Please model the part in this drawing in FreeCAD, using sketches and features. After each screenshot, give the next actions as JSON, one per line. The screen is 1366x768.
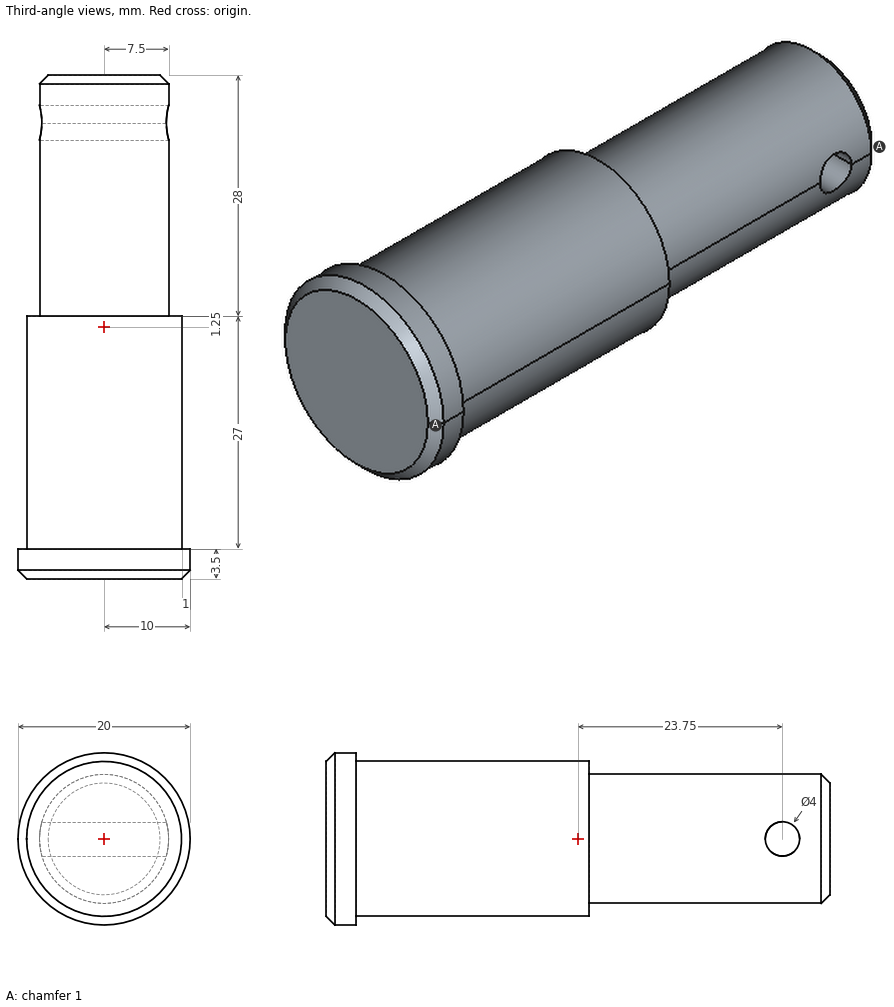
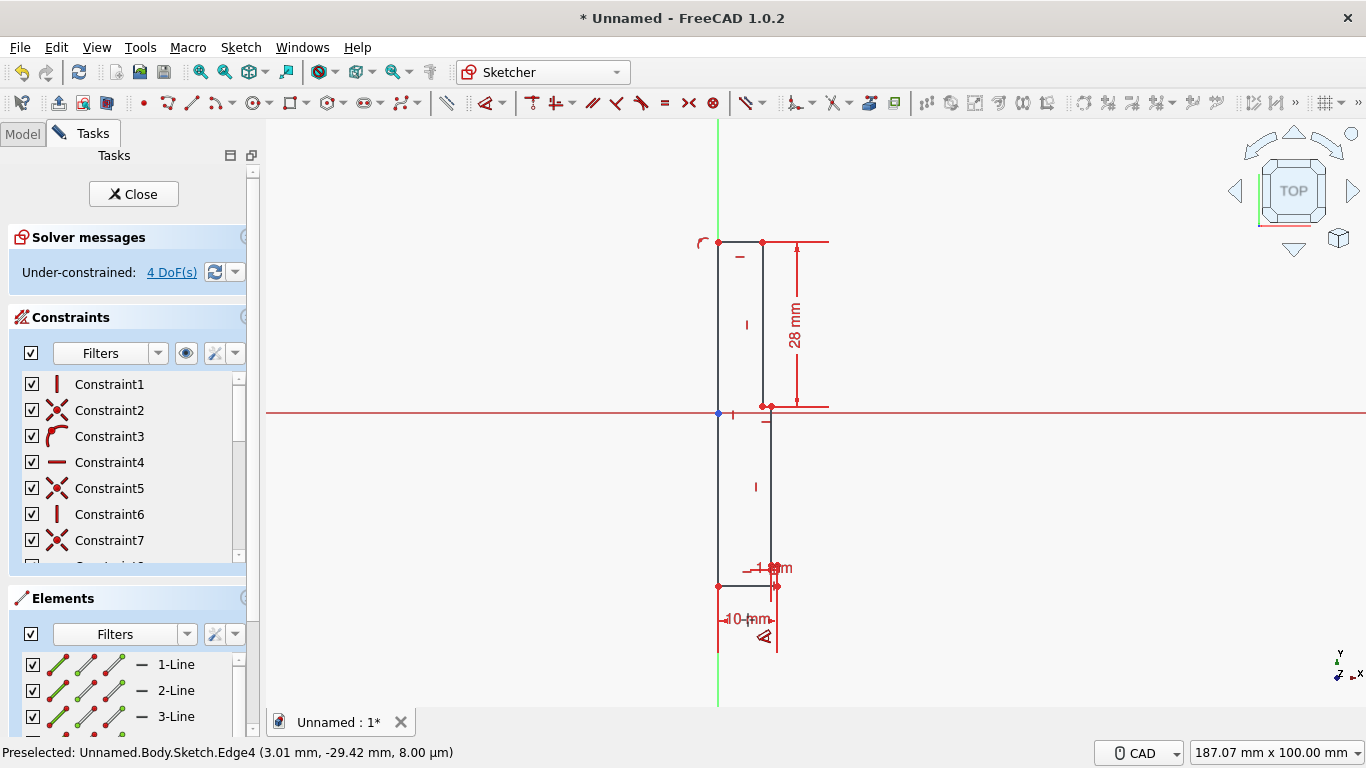
{"action": "left_click", "coordinate": [771, 518]}
{"action": "left_click", "coordinate": [805, 486]}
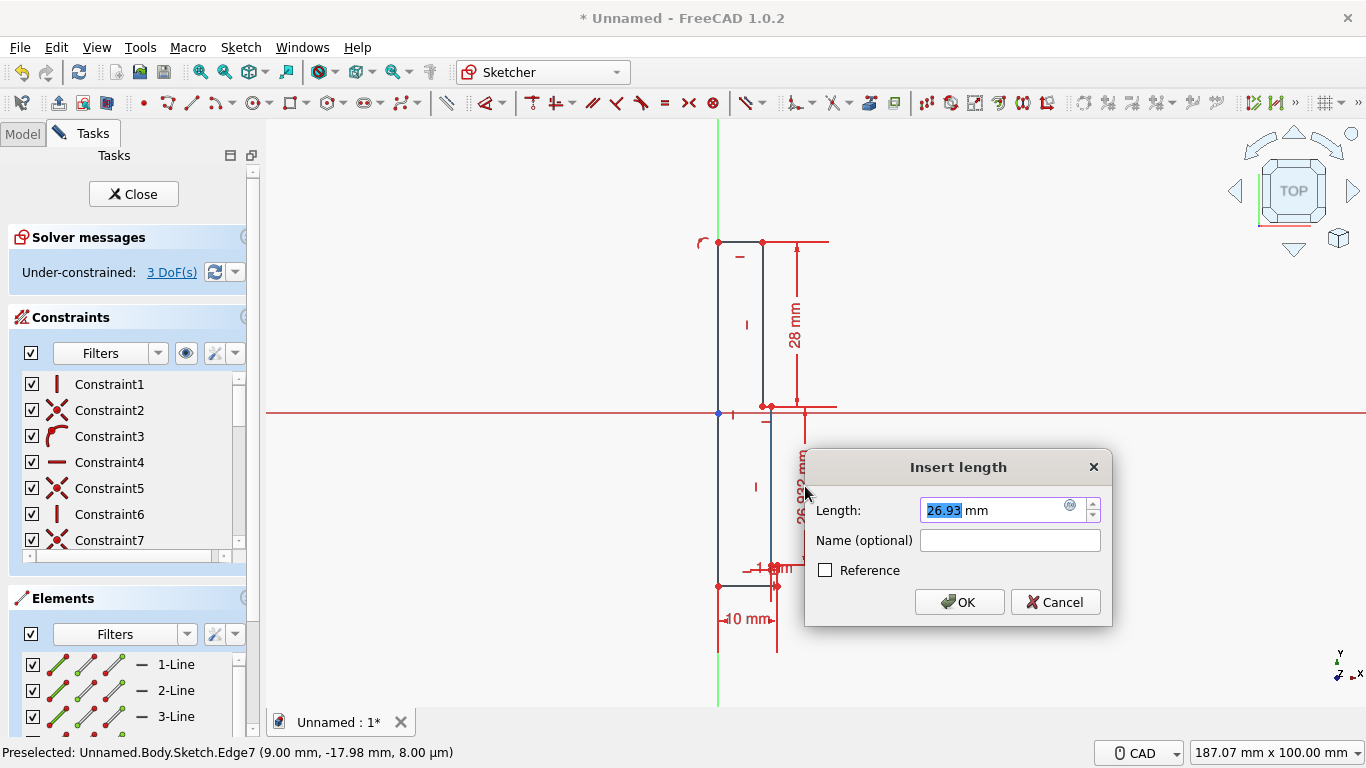
{"action": "type", "text": "27"}
{"action": "key", "text": "Return"}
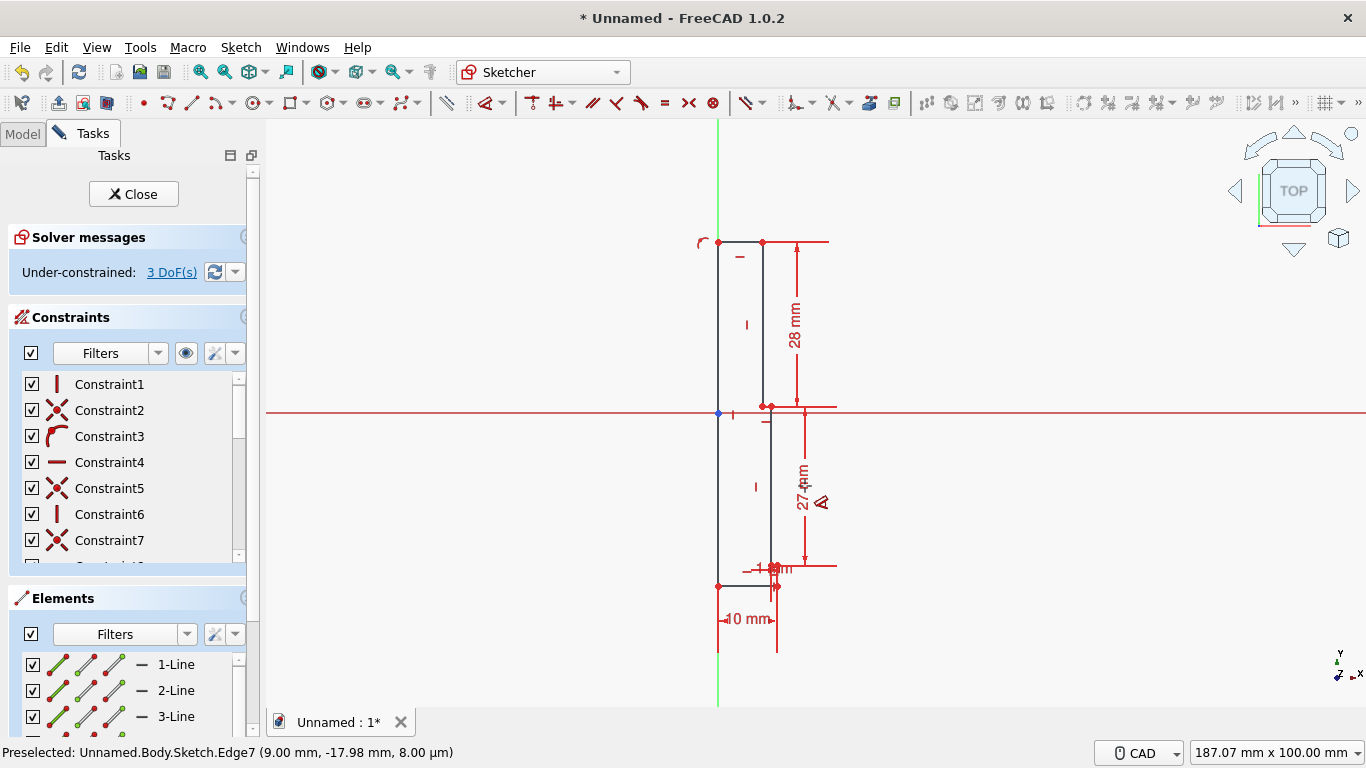
{"action": "left_click", "coordinate": [749, 242]}
{"action": "left_click", "coordinate": [740, 208]}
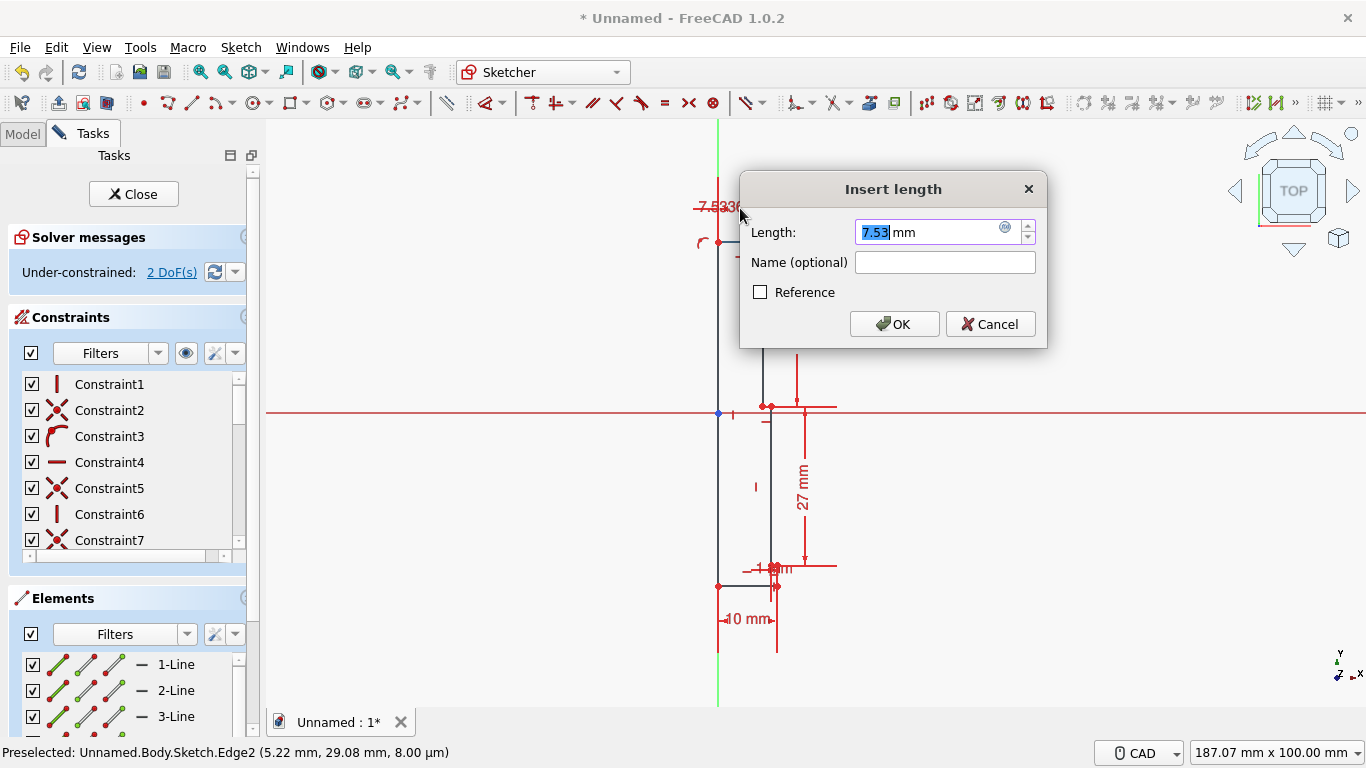
{"action": "type", "text": "7.5"}
{"action": "key", "text": "Return"}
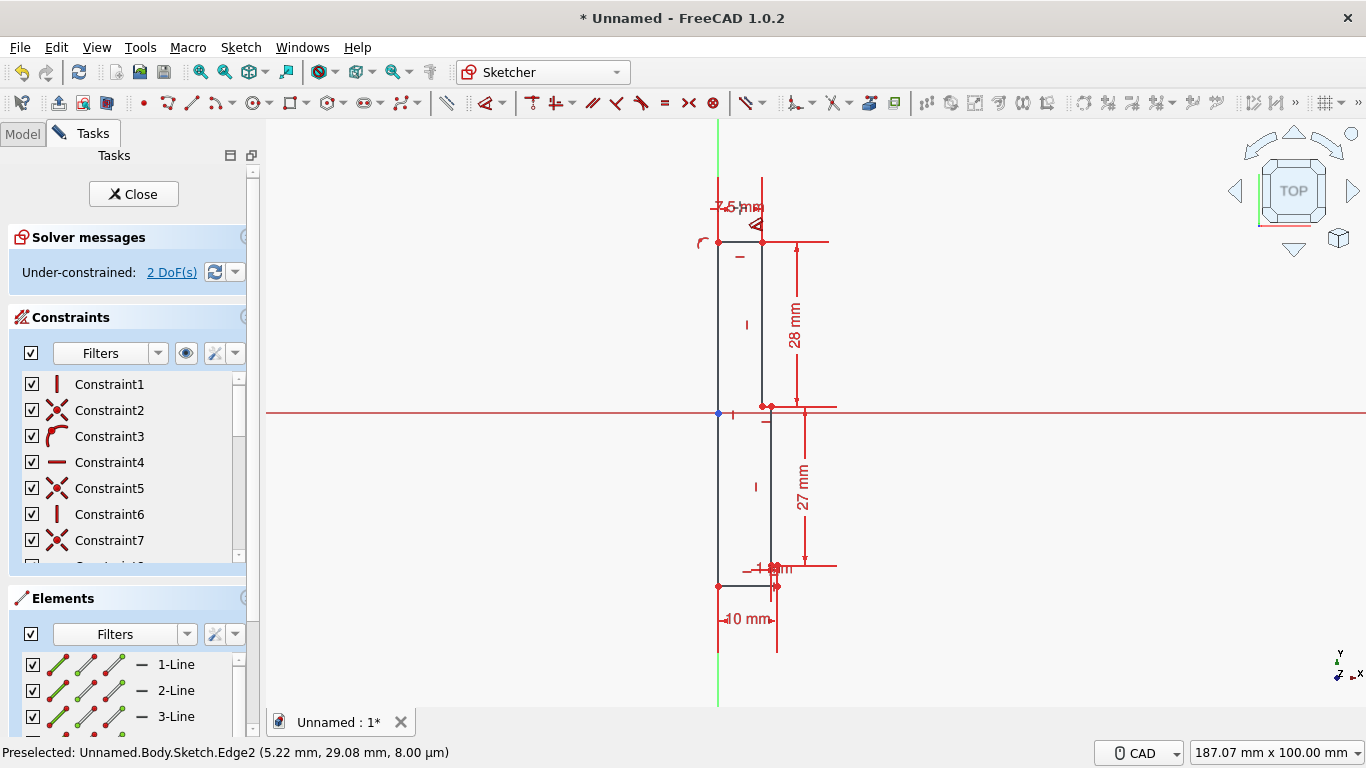
{"action": "scroll", "coordinate": [777, 576], "scroll_direction": "up", "scroll_amount": 4}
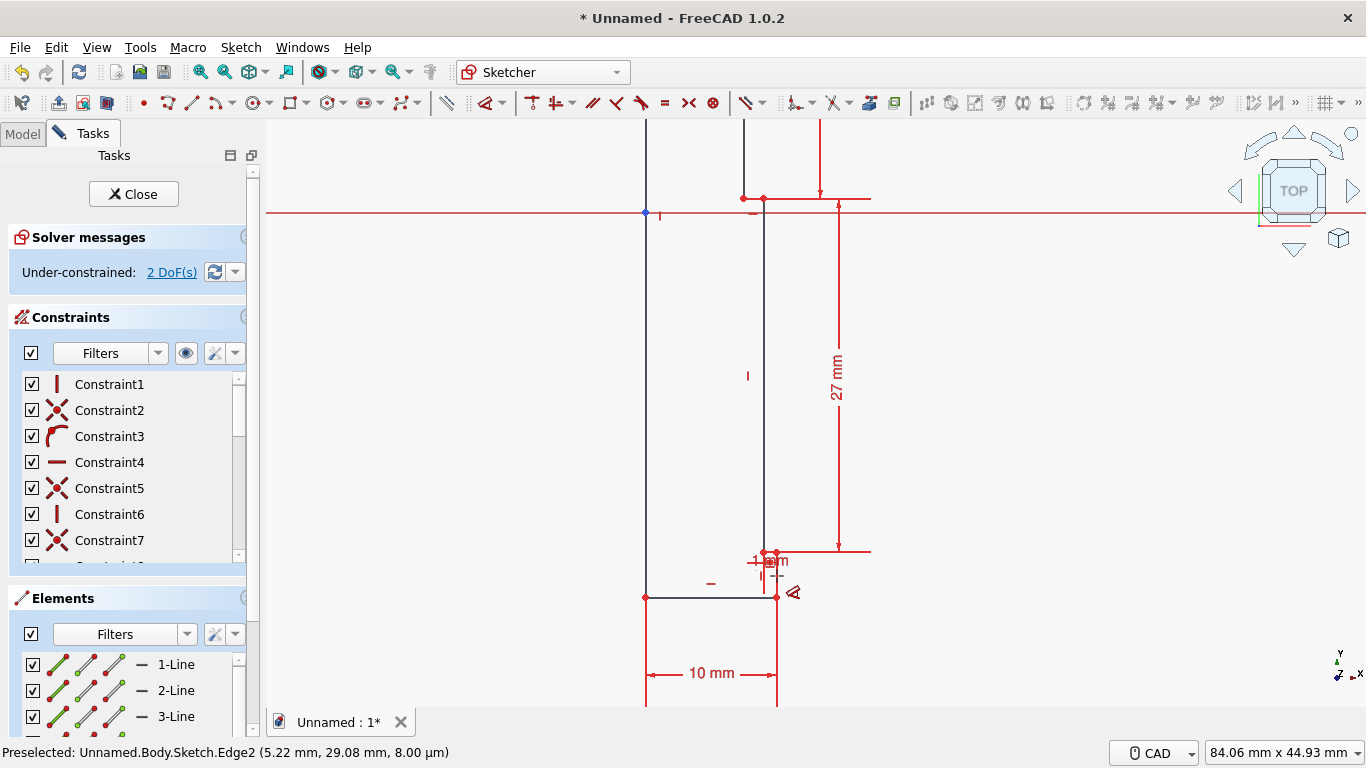
{"action": "left_click", "coordinate": [777, 575]}
{"action": "left_click", "coordinate": [811, 586]}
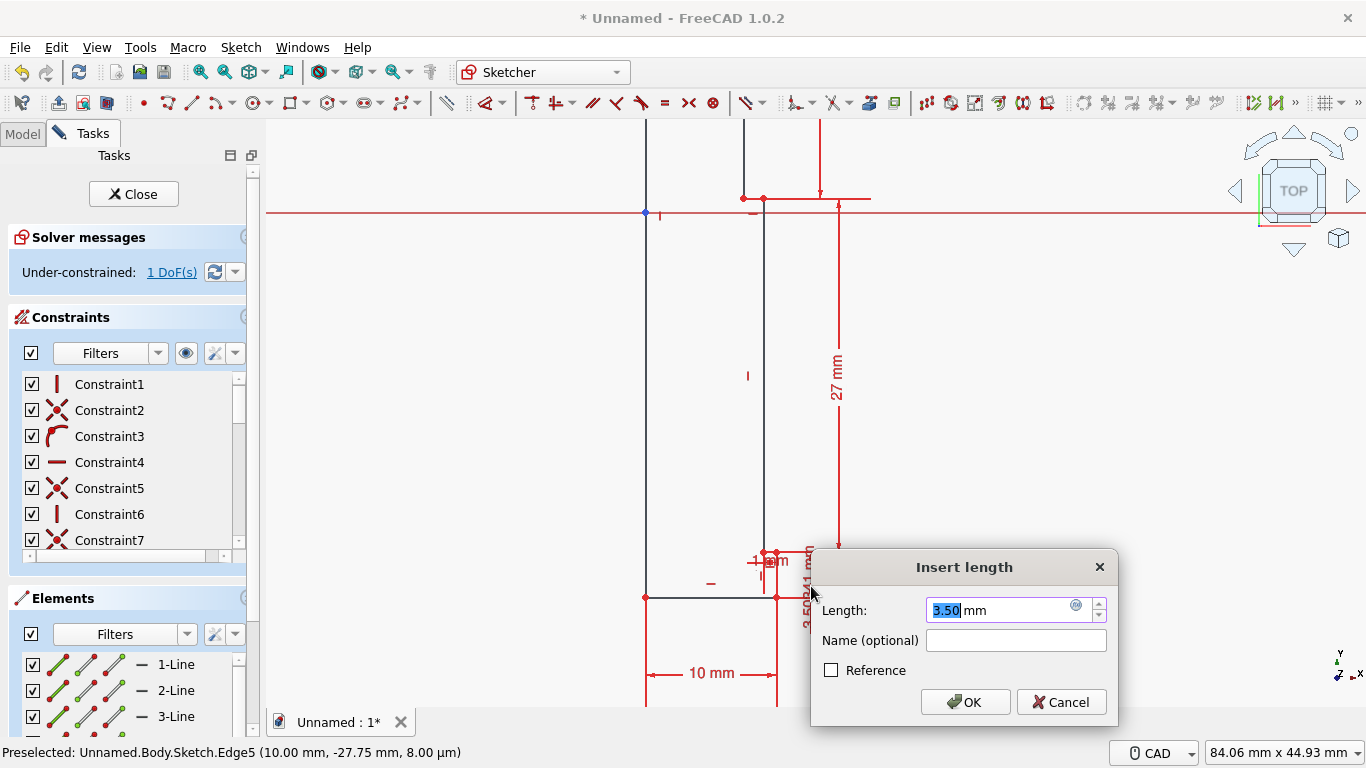
{"action": "type", "text": "3.5"}
{"action": "key", "text": "Return"}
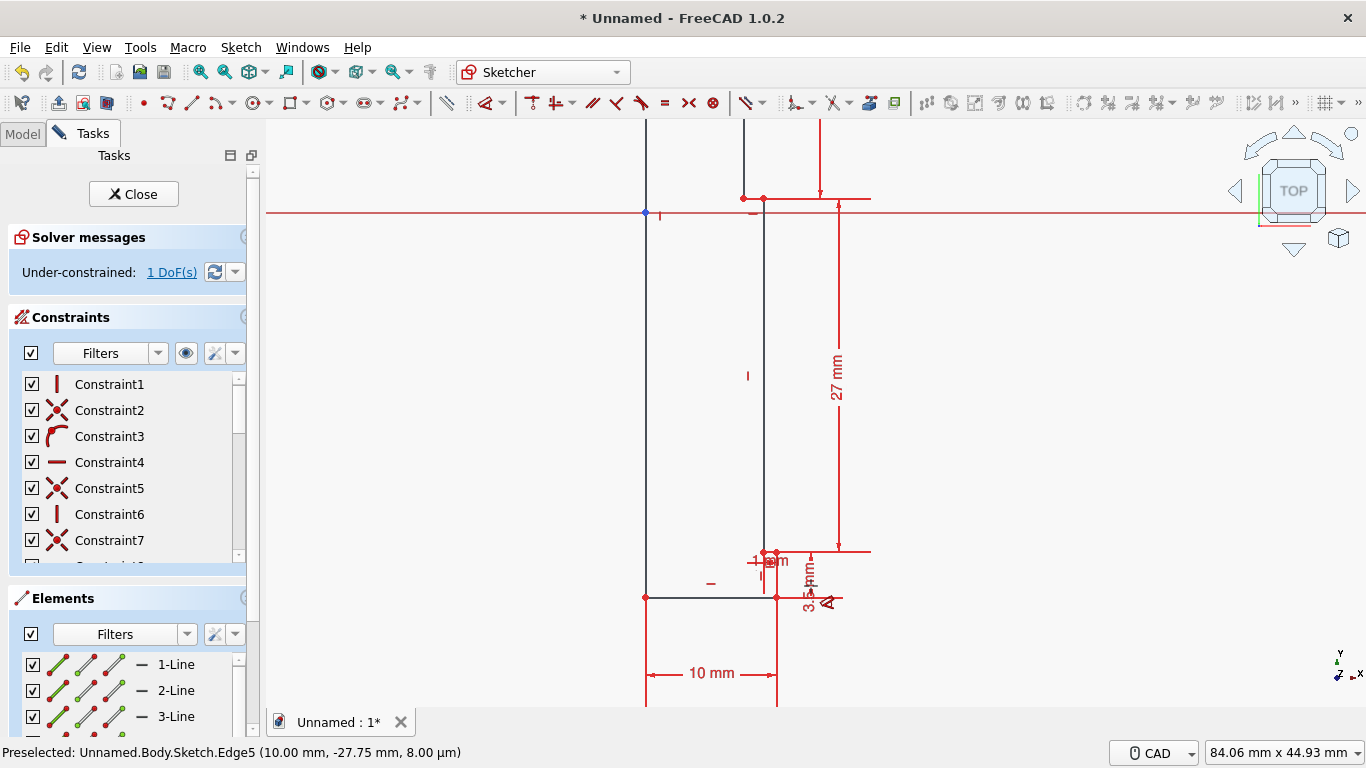
{"action": "scroll", "coordinate": [744, 199], "scroll_direction": "up", "scroll_amount": 5}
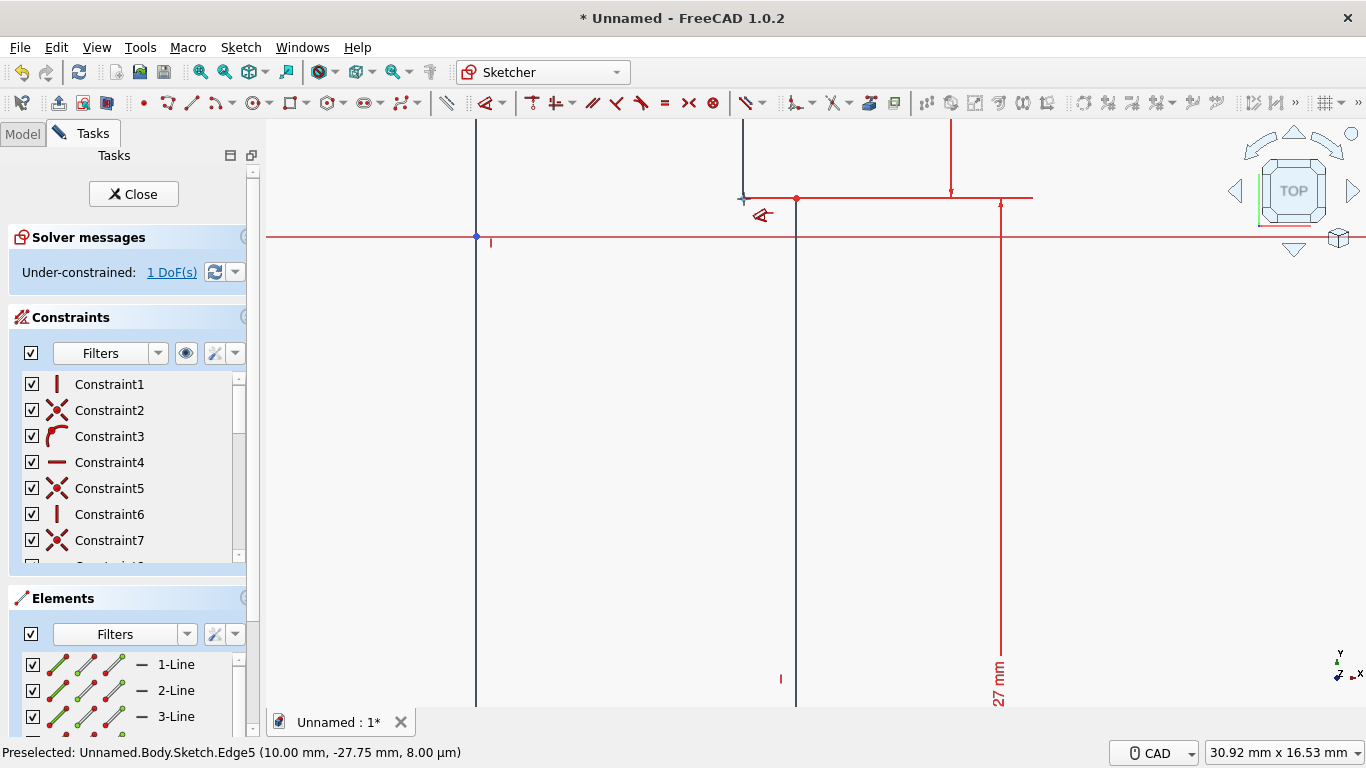
{"action": "left_click", "coordinate": [743, 198]}
{"action": "left_click", "coordinate": [442, 217]}